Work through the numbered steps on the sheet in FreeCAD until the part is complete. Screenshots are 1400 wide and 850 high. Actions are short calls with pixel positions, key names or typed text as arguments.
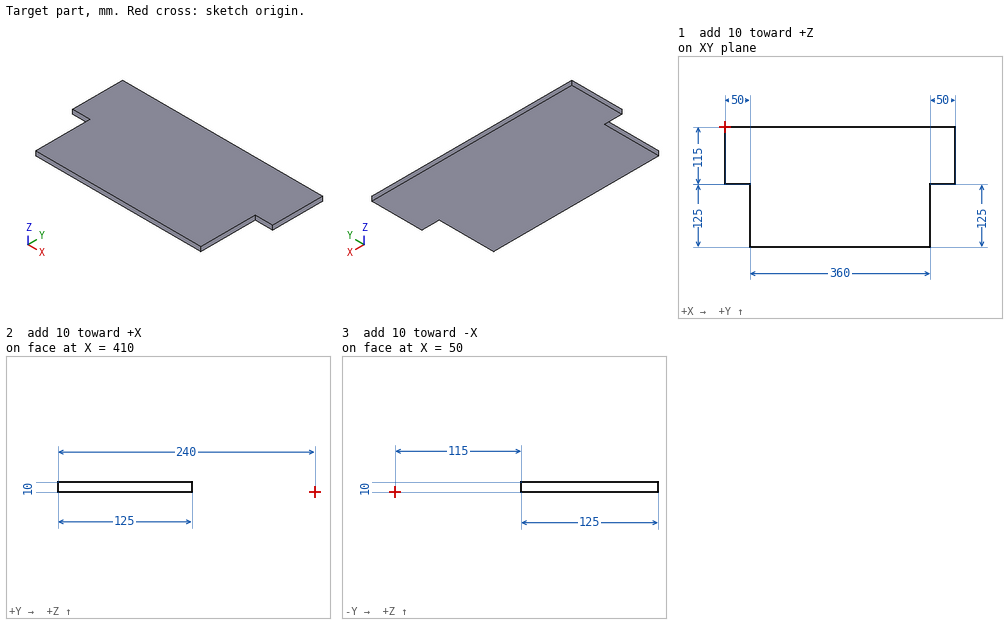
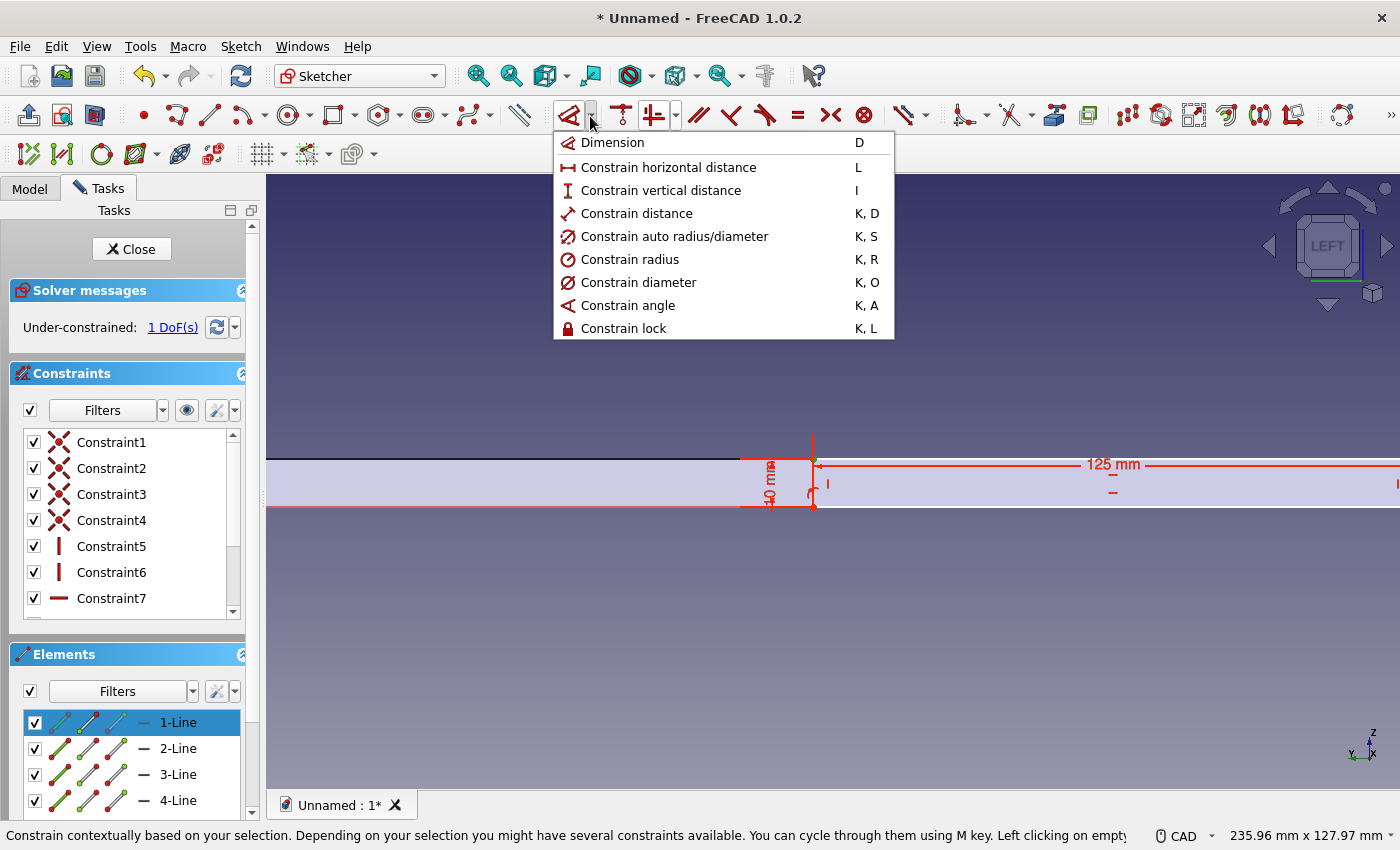
click(724, 168)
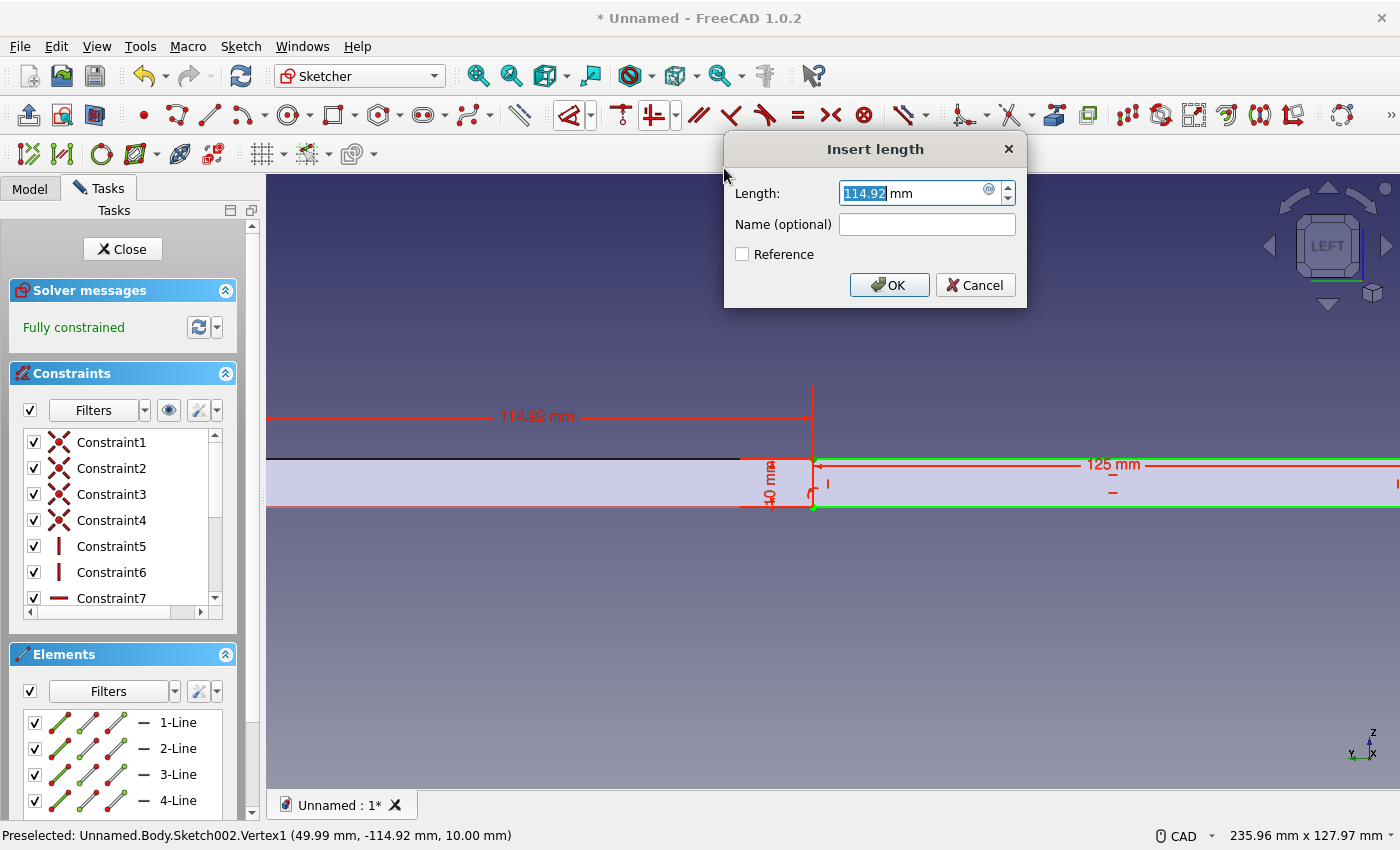
text(115)
key(Return)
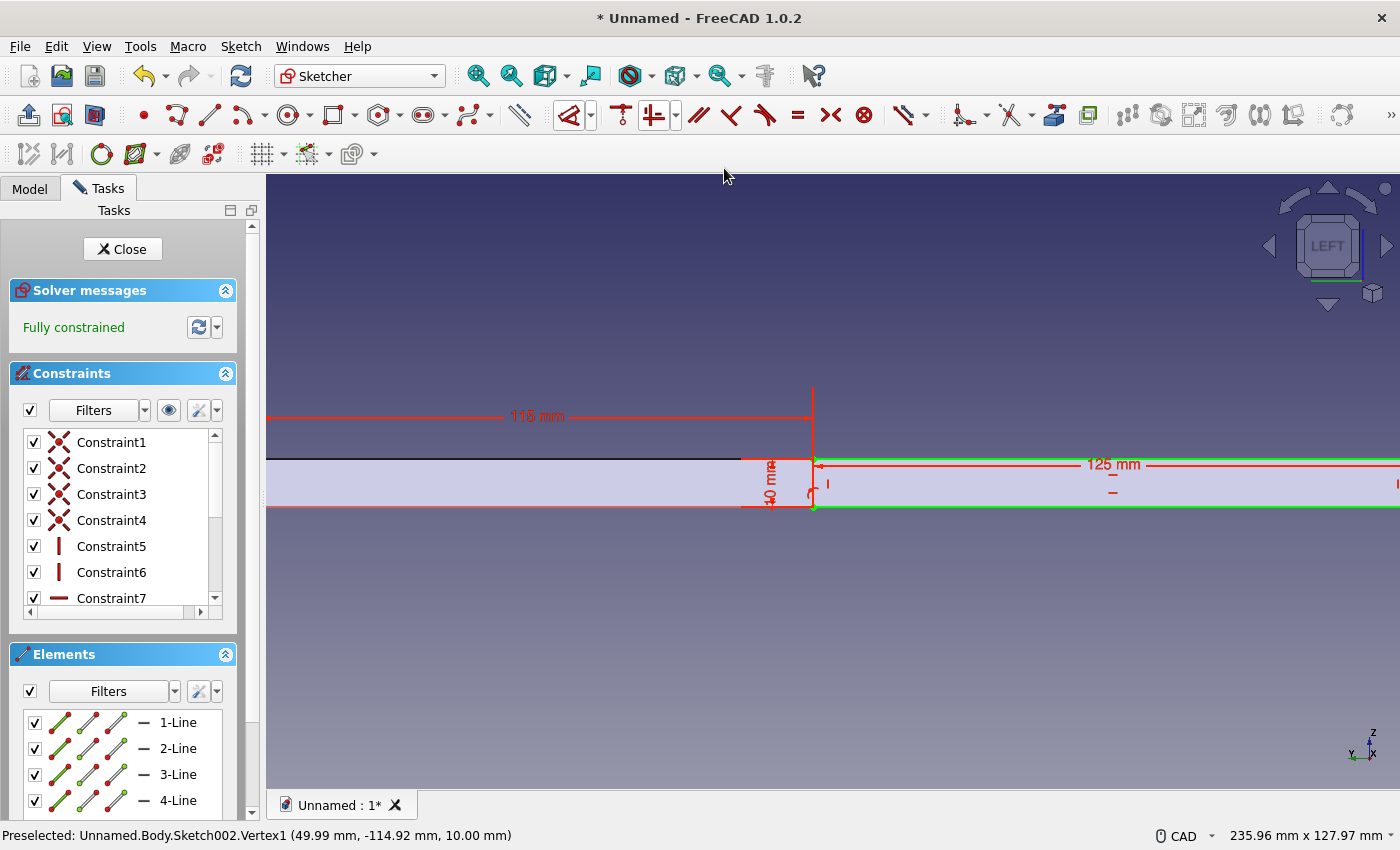
click(123, 249)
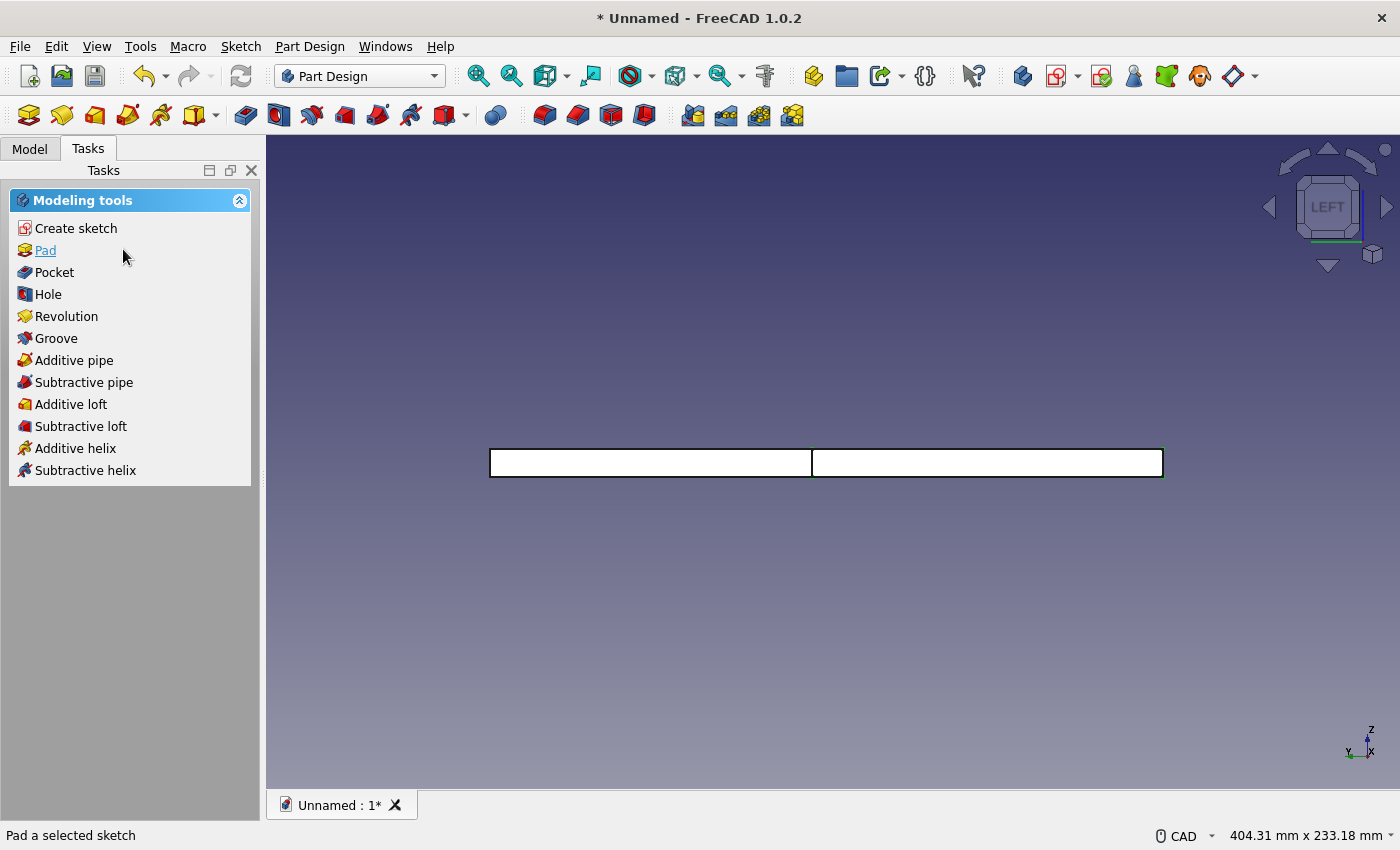
click(29, 116)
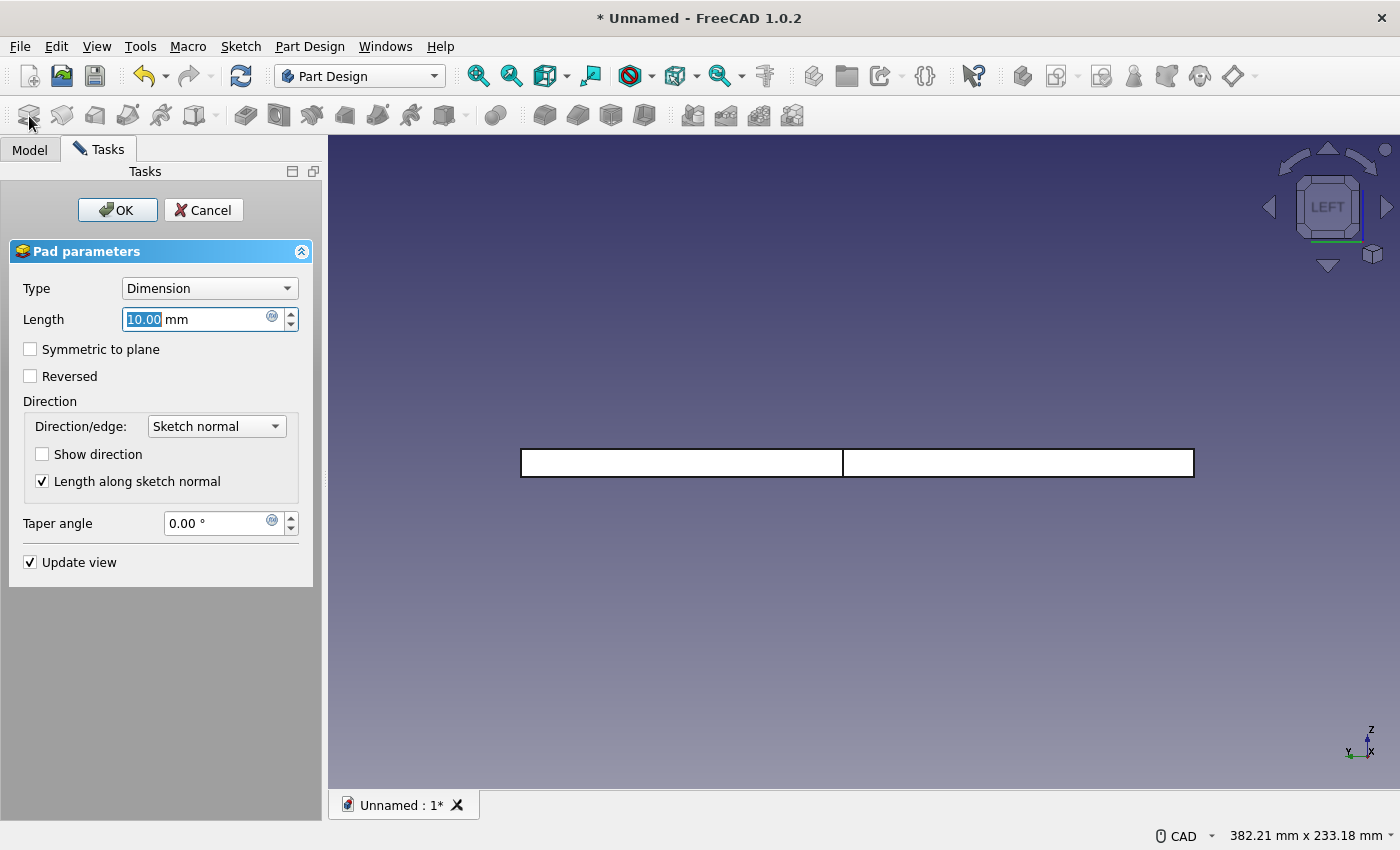
text(10)
key(Tab)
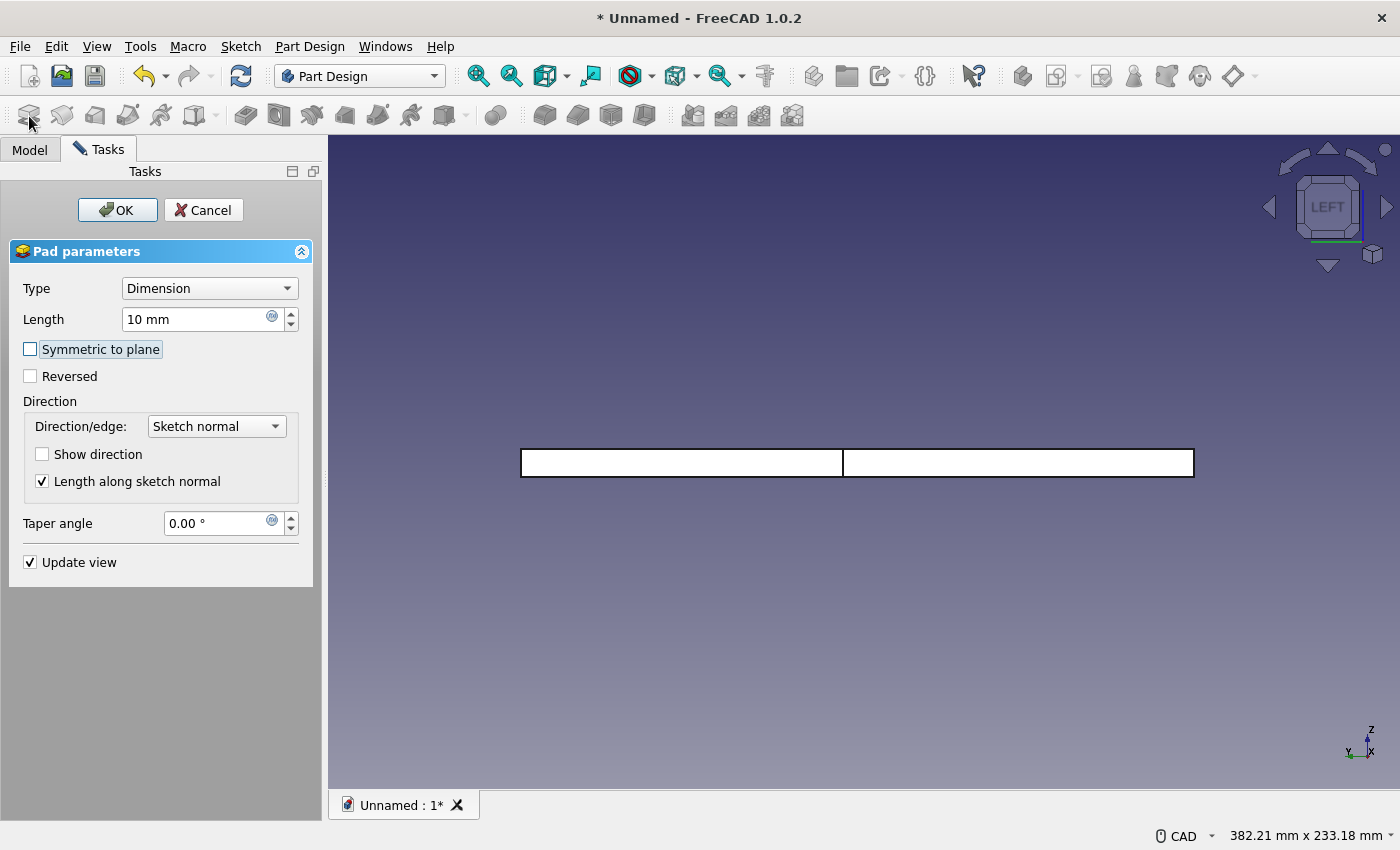
click(118, 210)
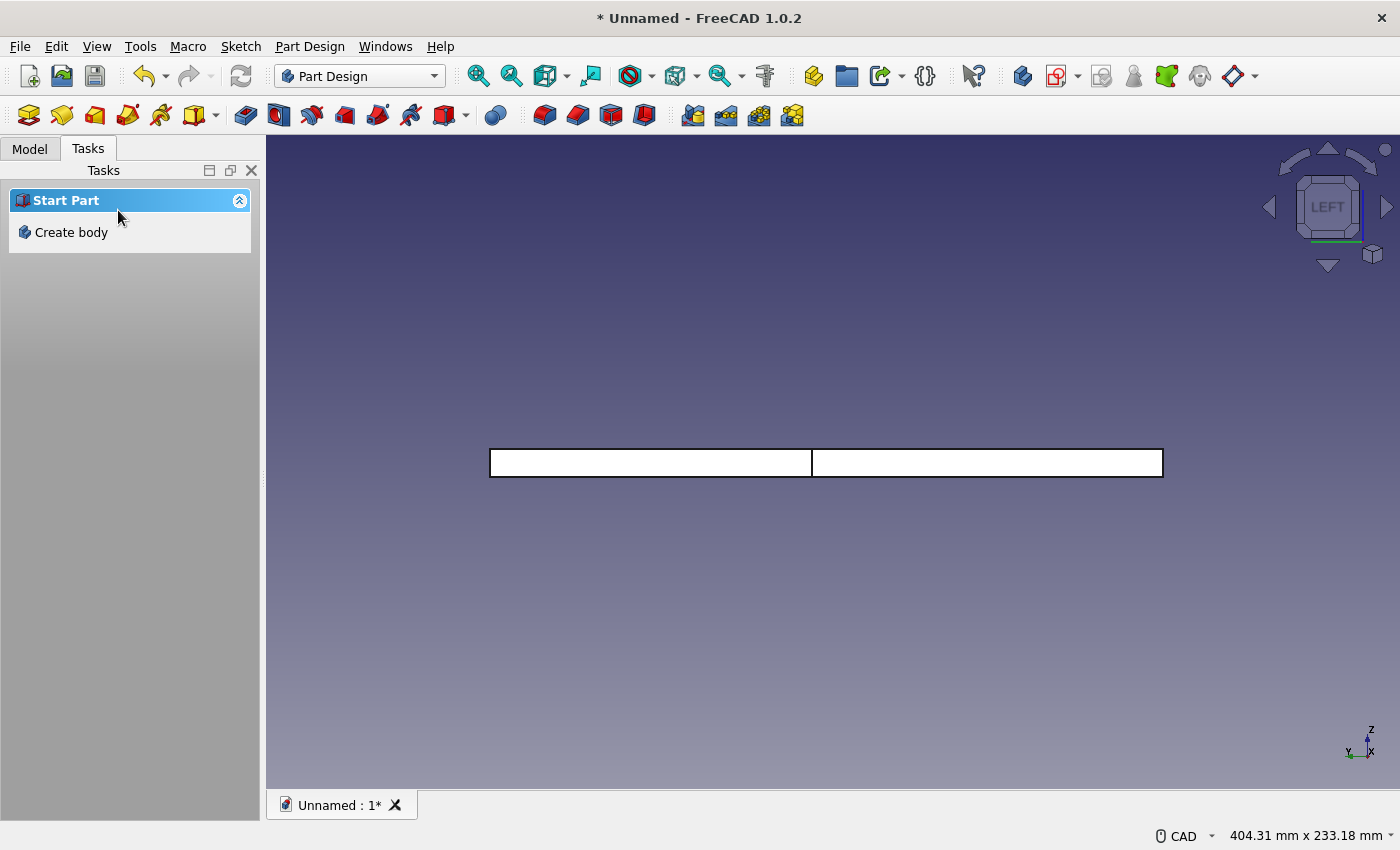
key(0)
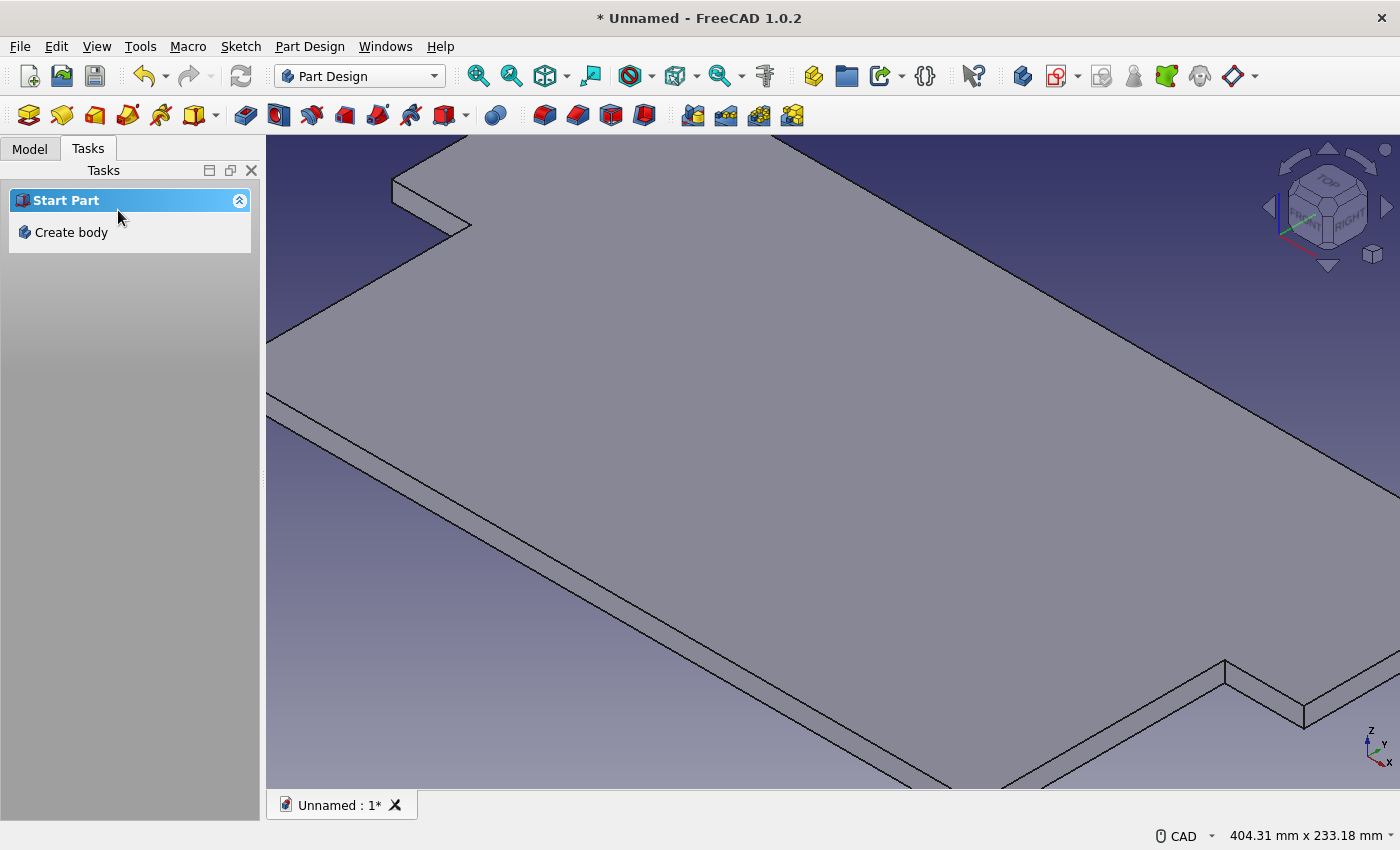
click(479, 76)